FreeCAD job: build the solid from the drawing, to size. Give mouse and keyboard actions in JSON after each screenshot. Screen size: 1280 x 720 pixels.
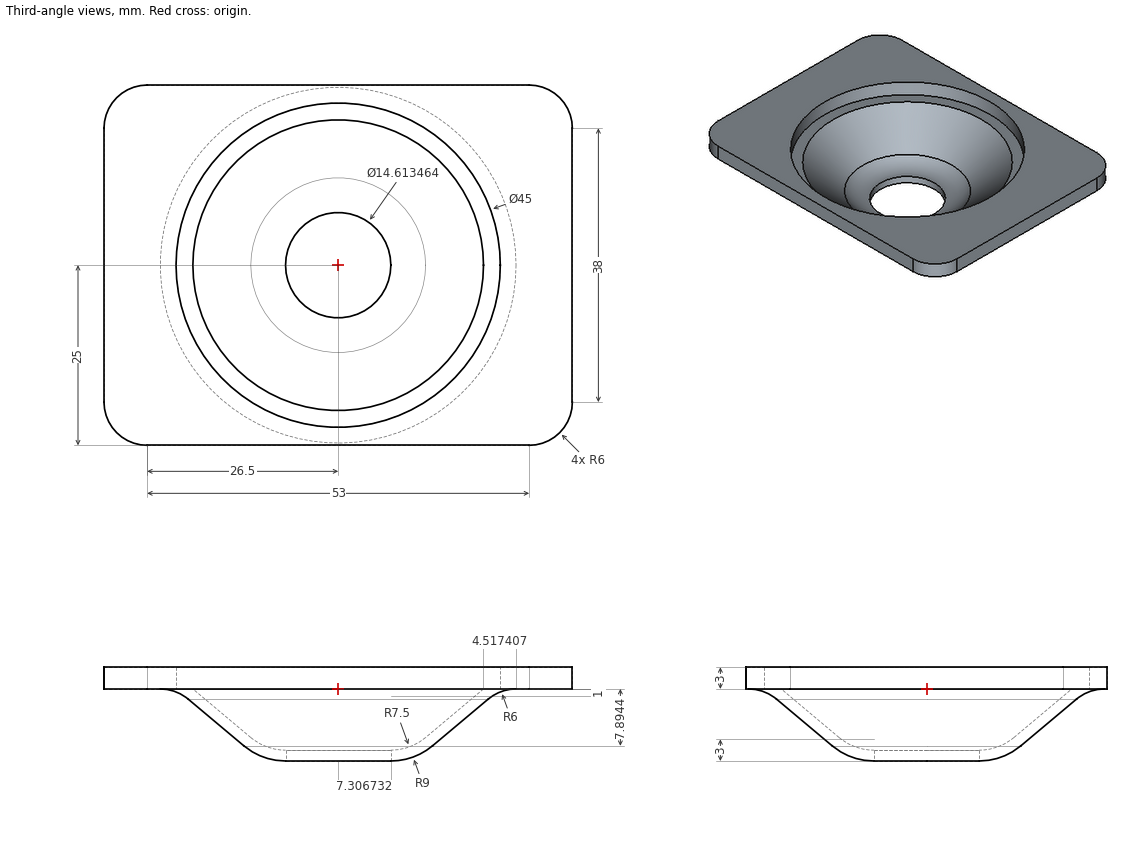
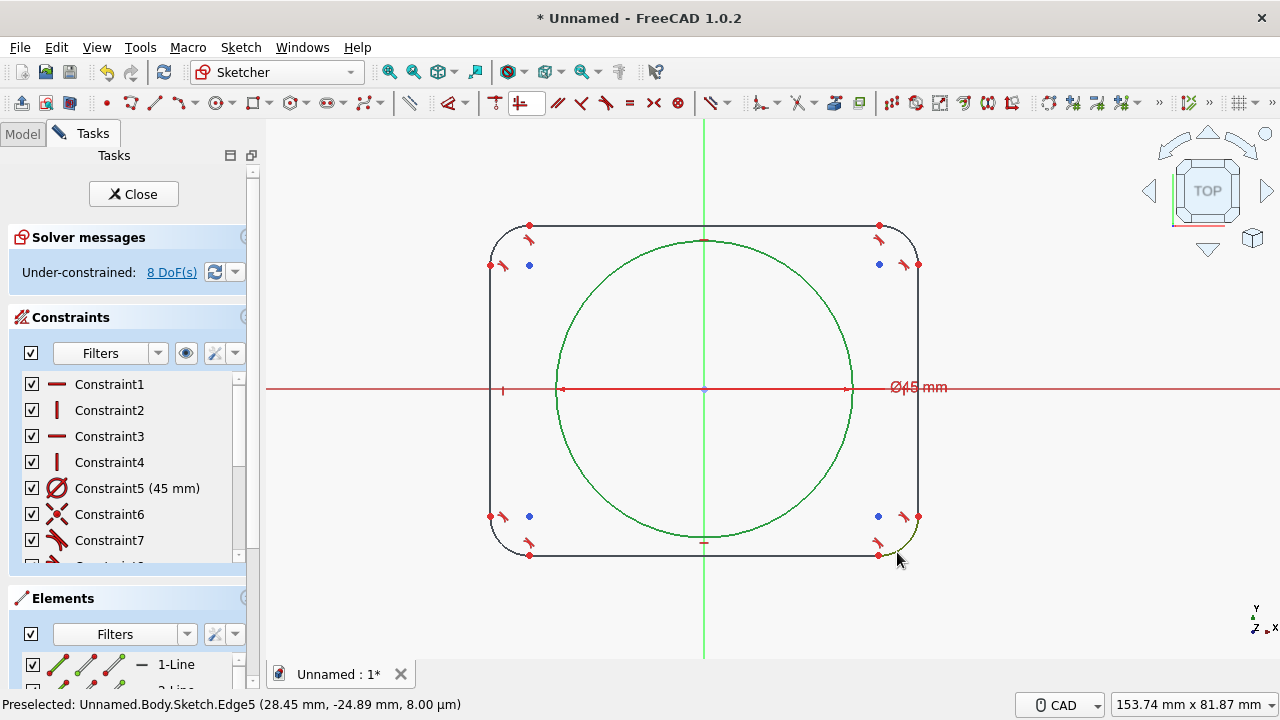
{"action": "left_click", "coordinate": [914, 247]}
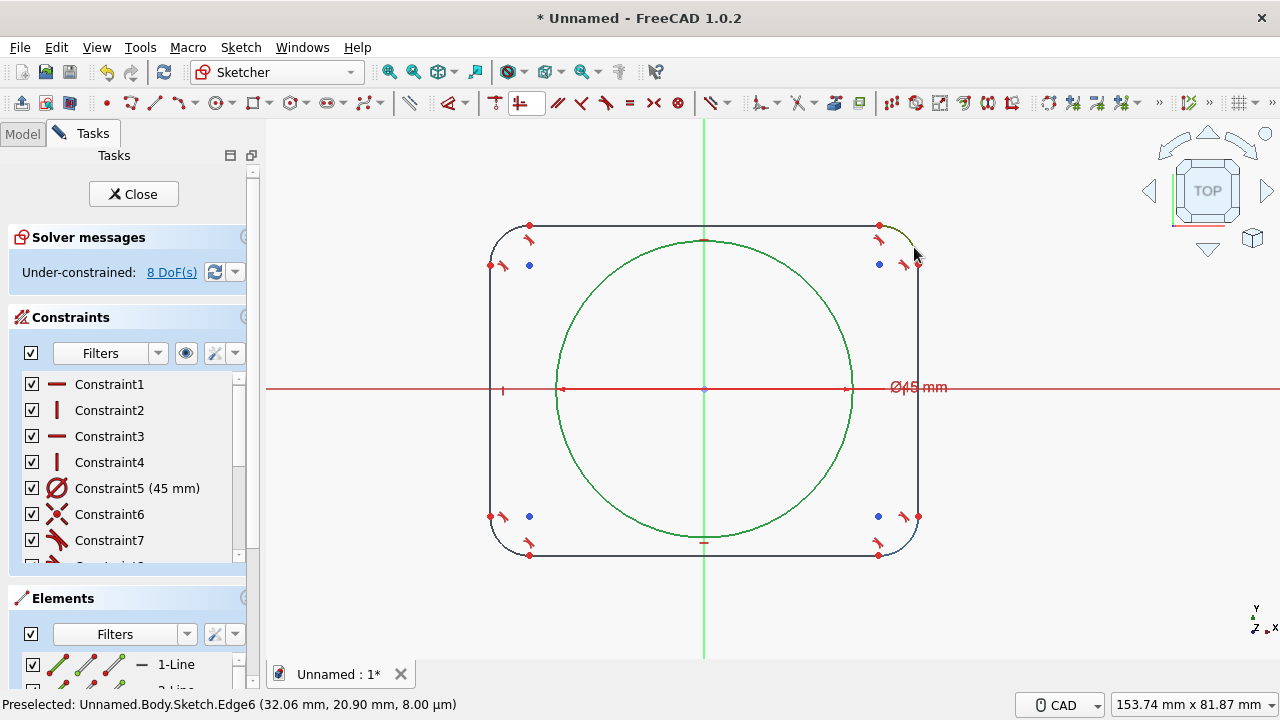
{"action": "left_click", "coordinate": [512, 230]}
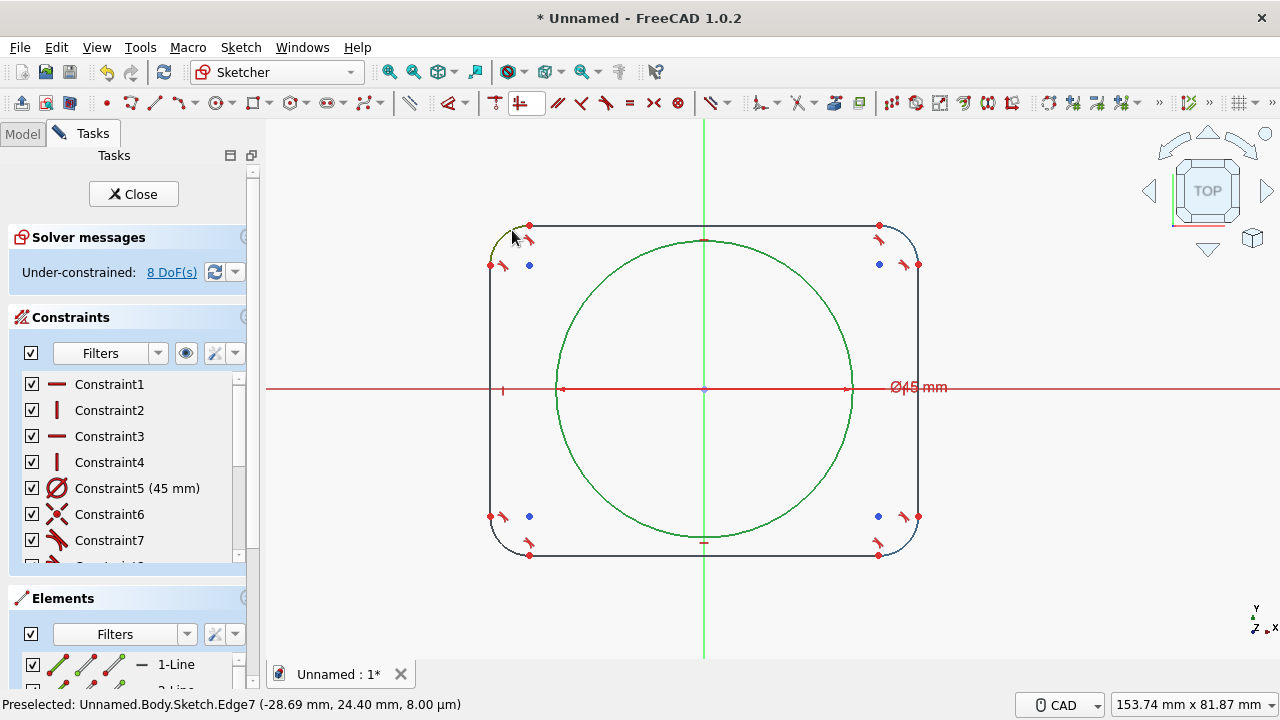
{"action": "left_click", "coordinate": [495, 534]}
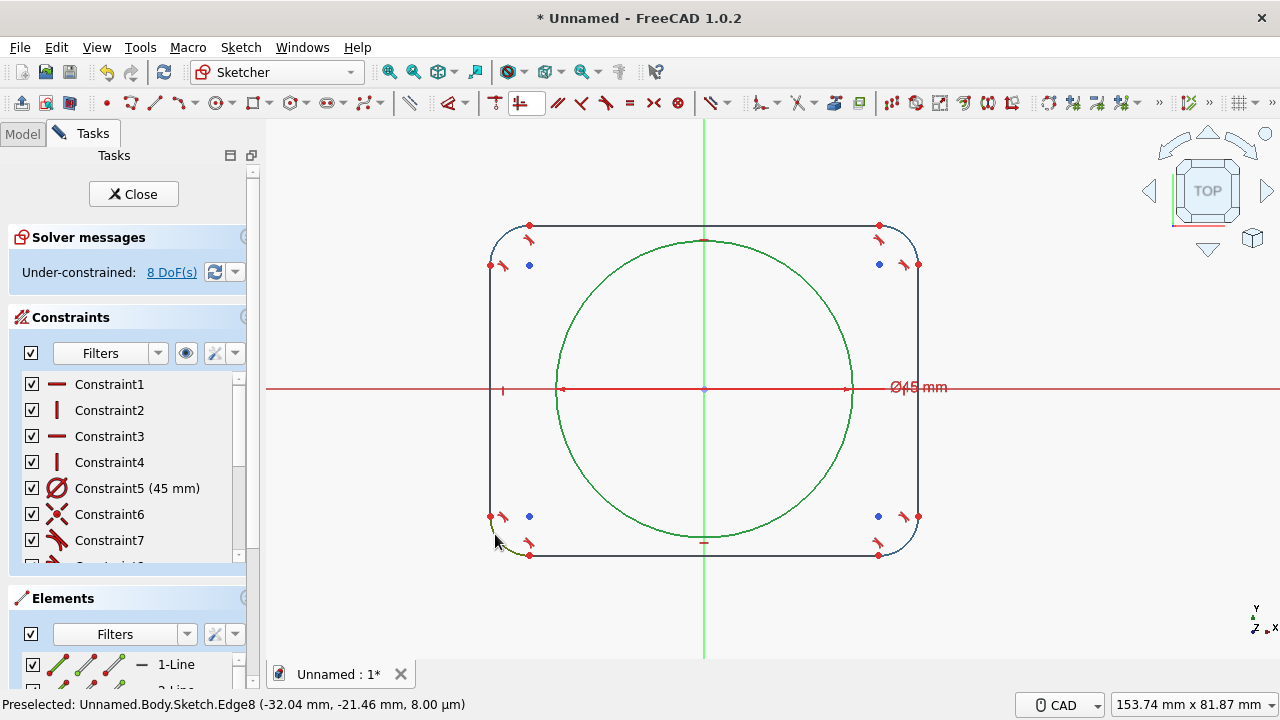
{"action": "key", "text": "e"}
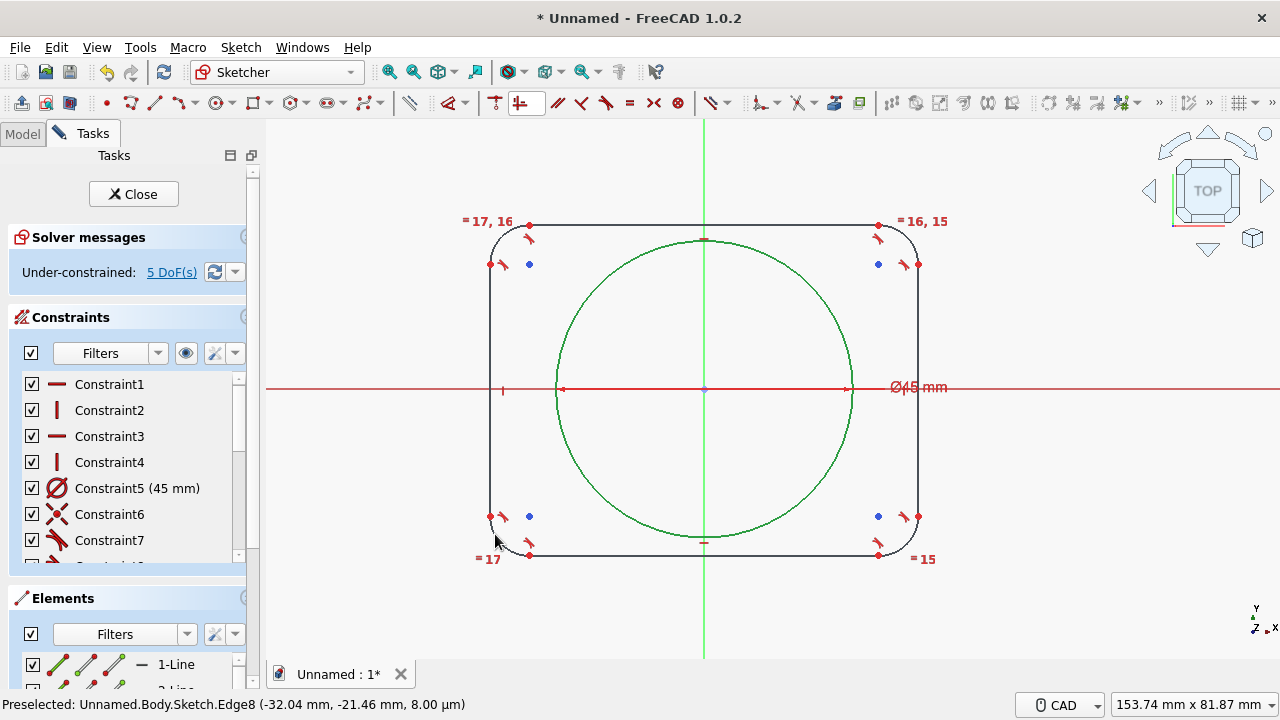
{"action": "key", "text": "d"}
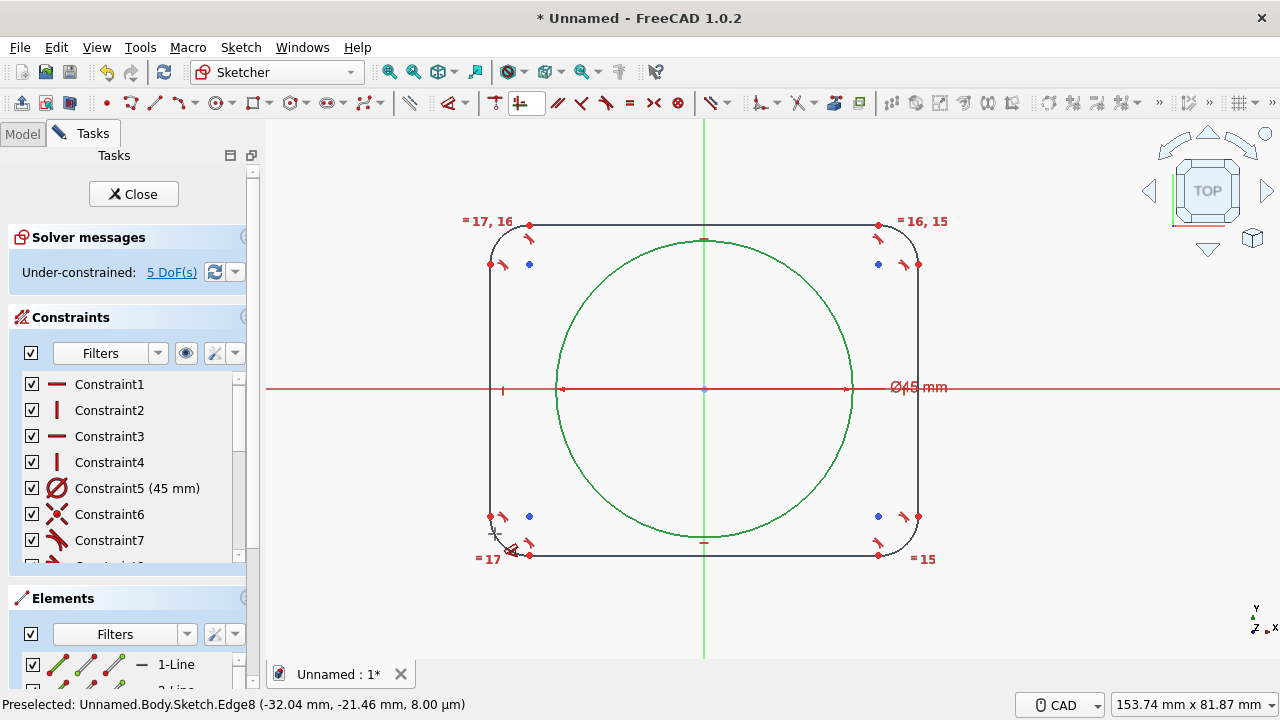
{"action": "left_click", "coordinate": [897, 552]}
{"action": "left_click", "coordinate": [912, 580]}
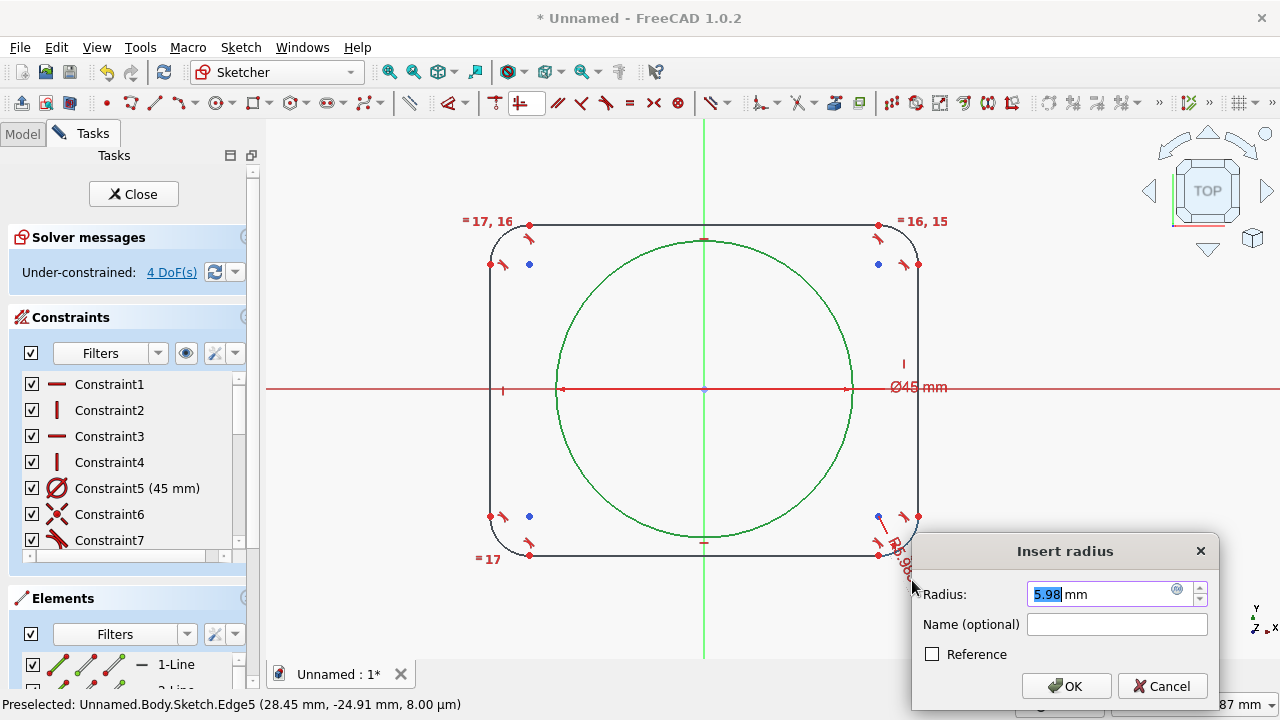
{"action": "type", "text": "6"}
{"action": "key", "text": "Return"}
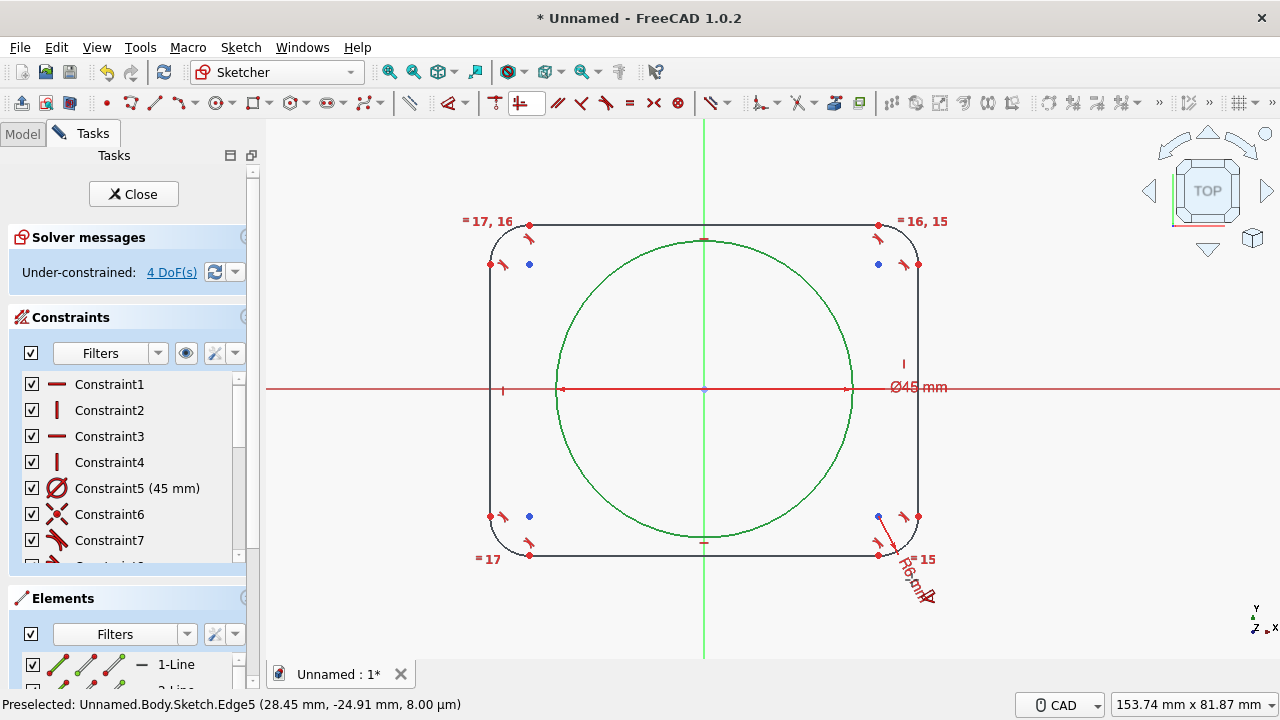
{"action": "left_click", "coordinate": [634, 556]}
{"action": "left_click", "coordinate": [624, 590]}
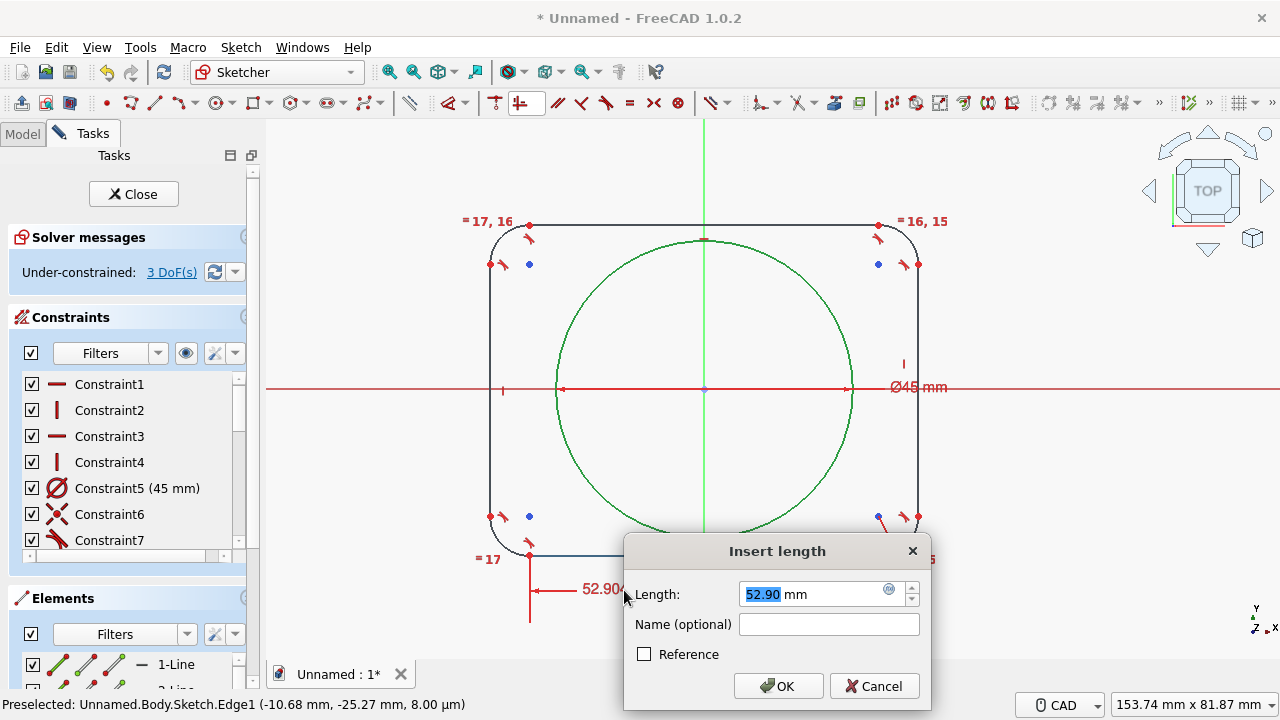
{"action": "type", "text": "53"}
{"action": "key", "text": "Return"}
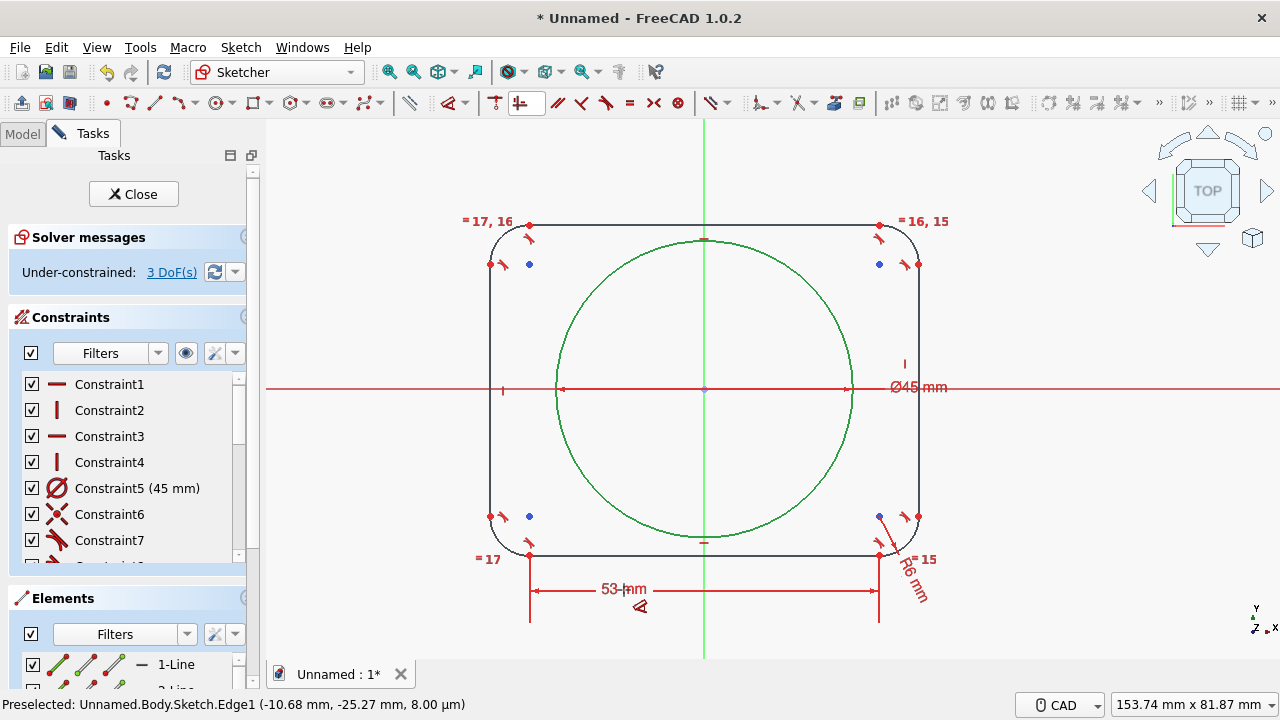
{"action": "left_click", "coordinate": [919, 441]}
{"action": "left_click", "coordinate": [953, 333]}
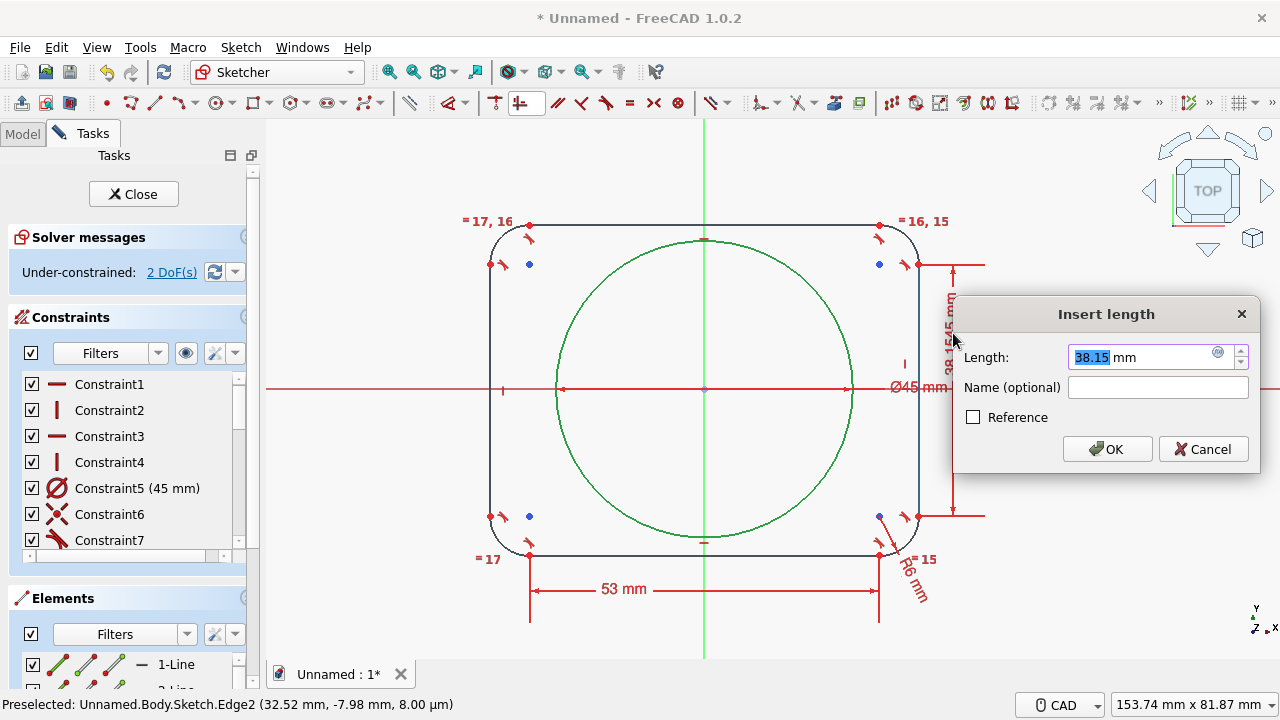
{"action": "type", "text": "38"}
{"action": "key", "text": "Return"}